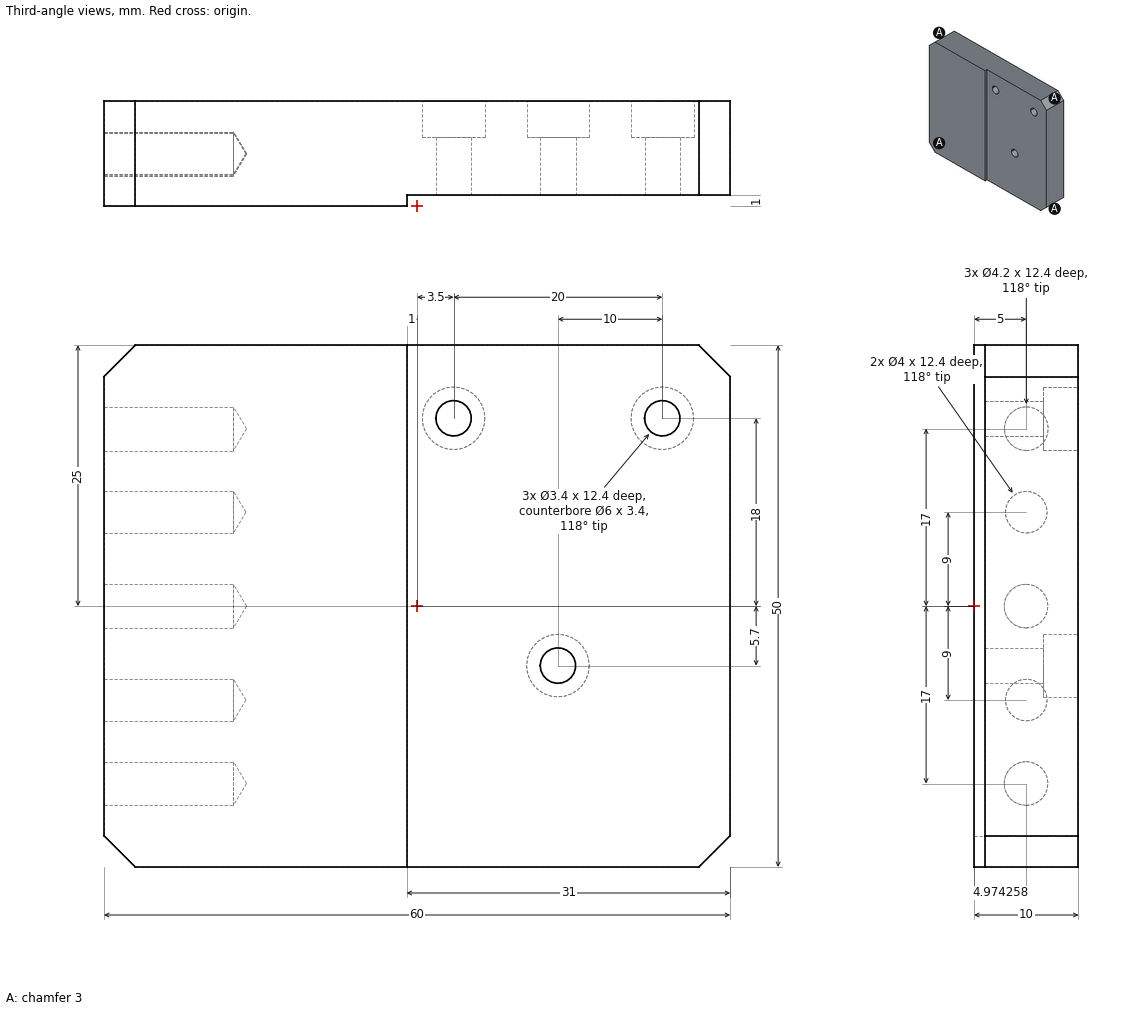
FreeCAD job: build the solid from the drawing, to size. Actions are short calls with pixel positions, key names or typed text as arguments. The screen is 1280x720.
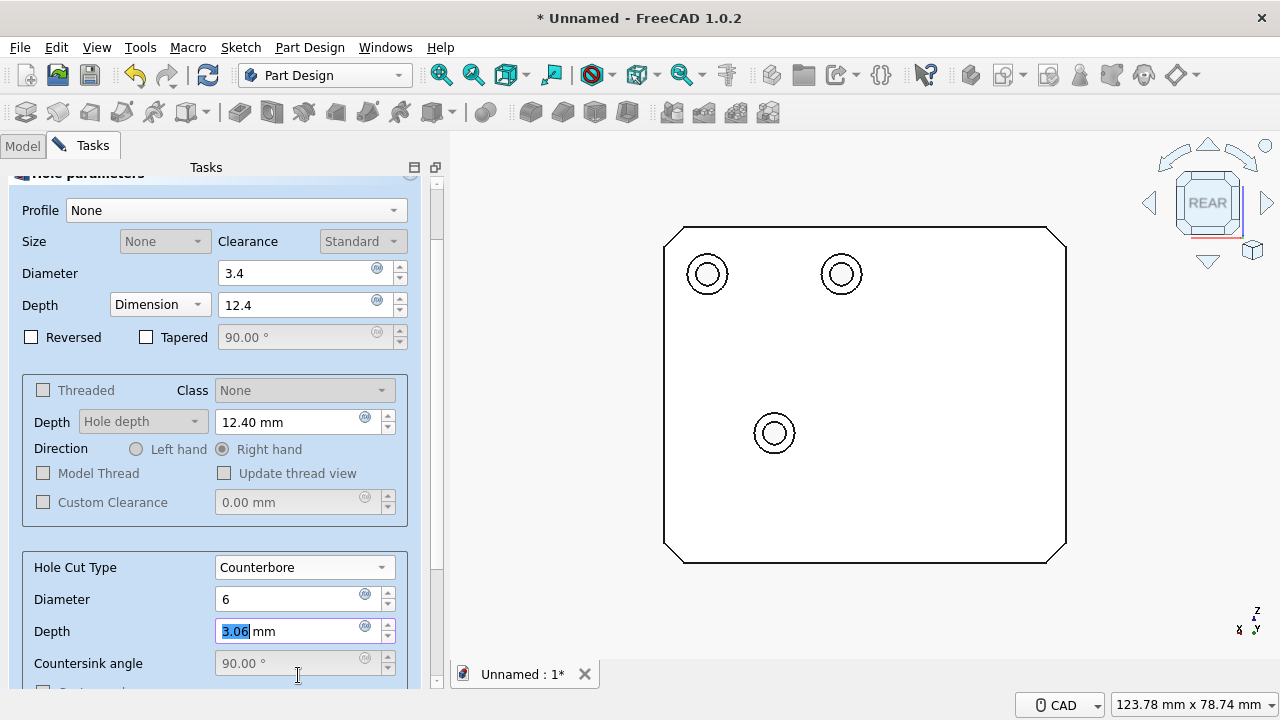
text(3.4)
key(Tab)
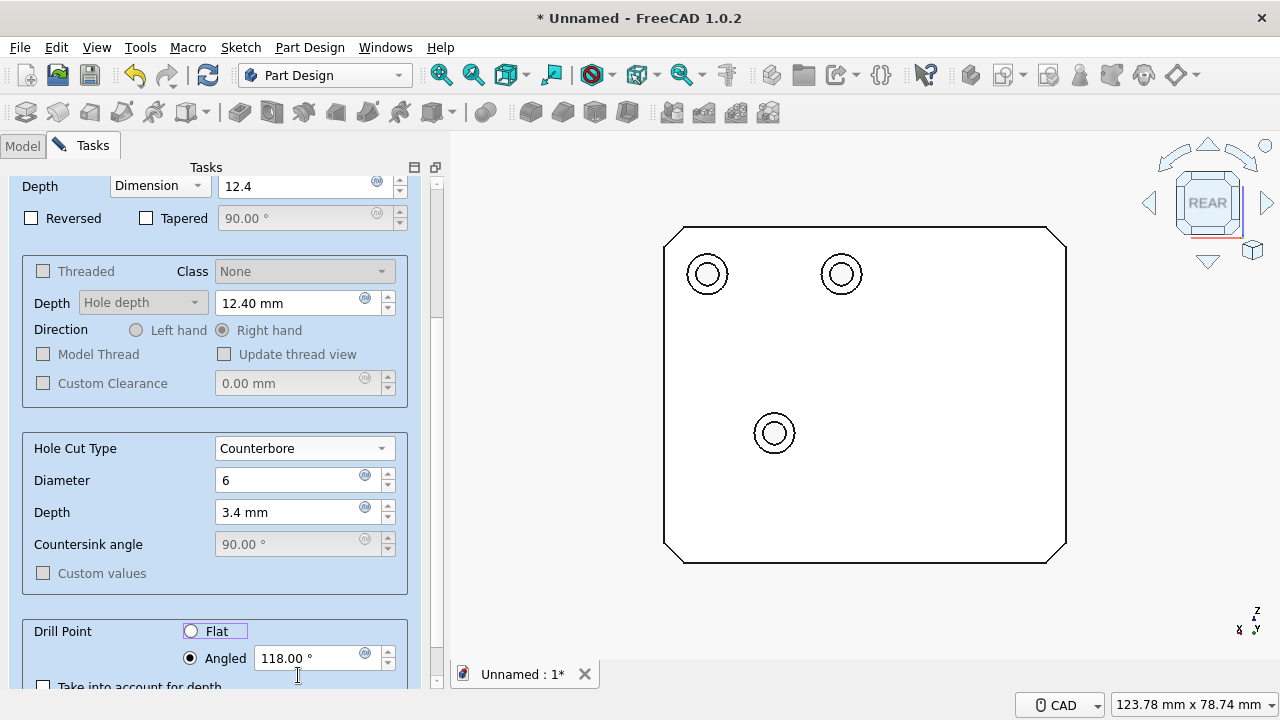
scroll(437, 432, up, 4)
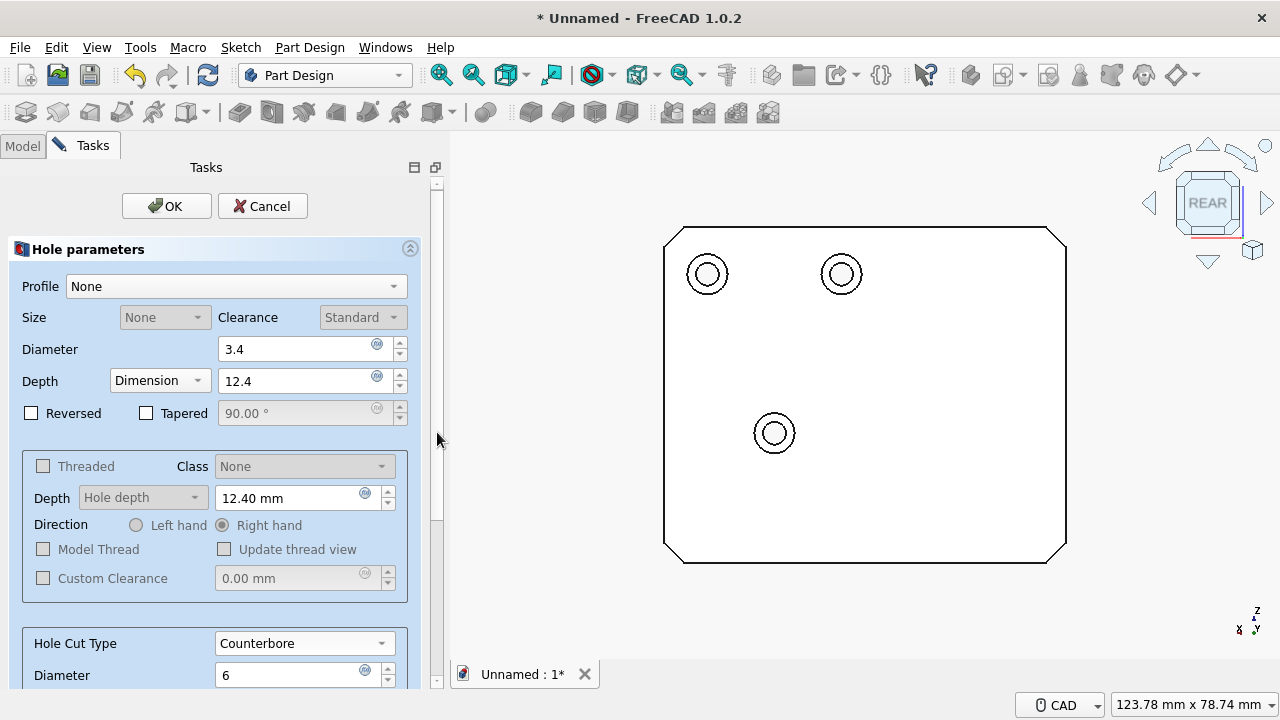
click(167, 206)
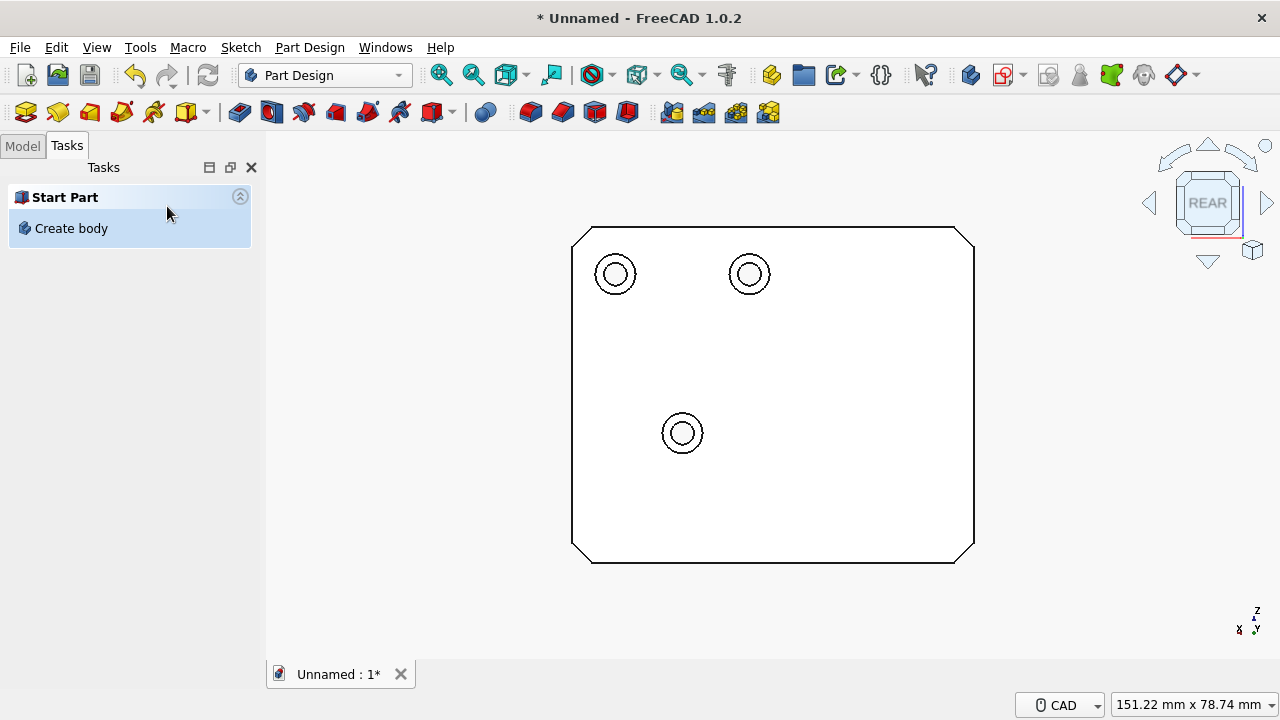
key(6)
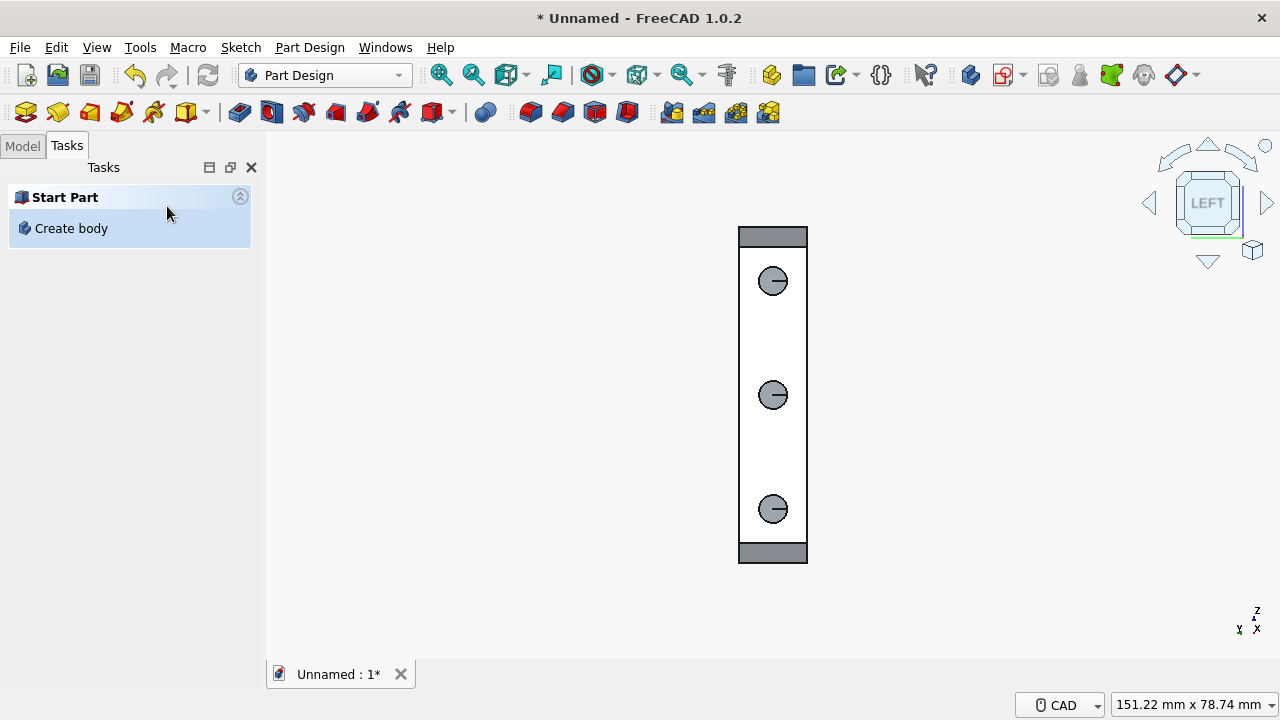
click(773, 436)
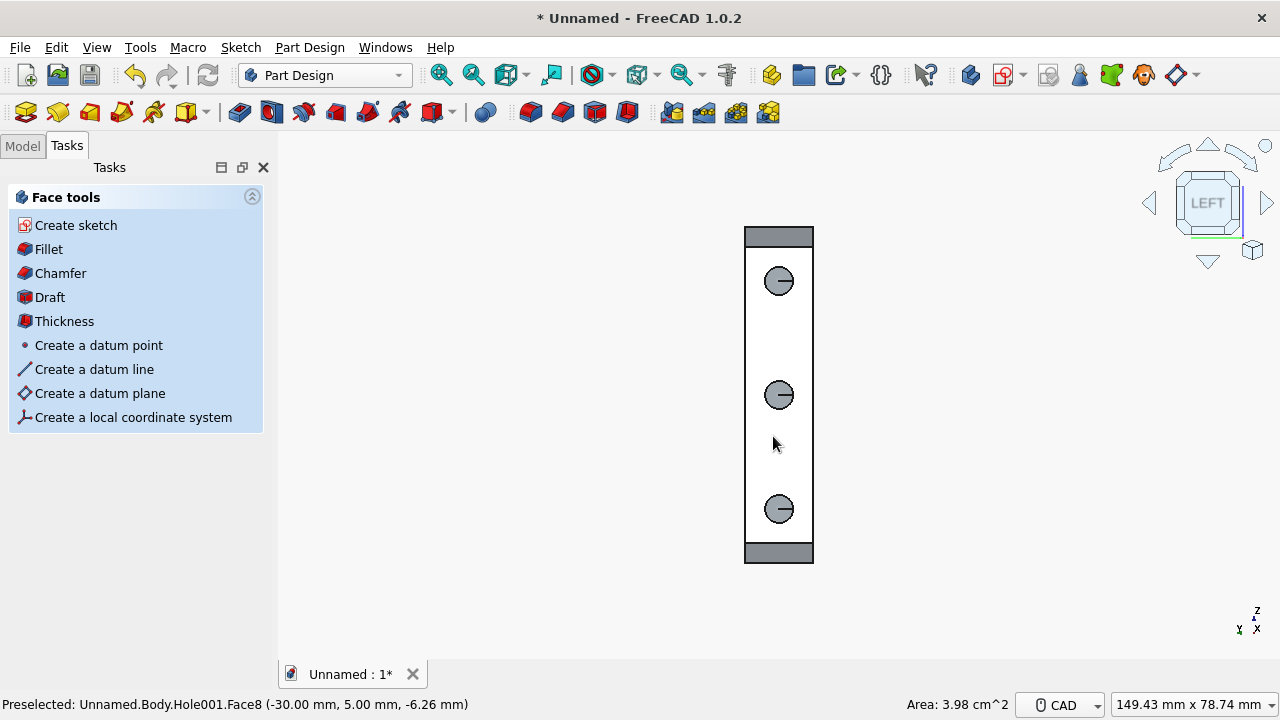
click(1004, 76)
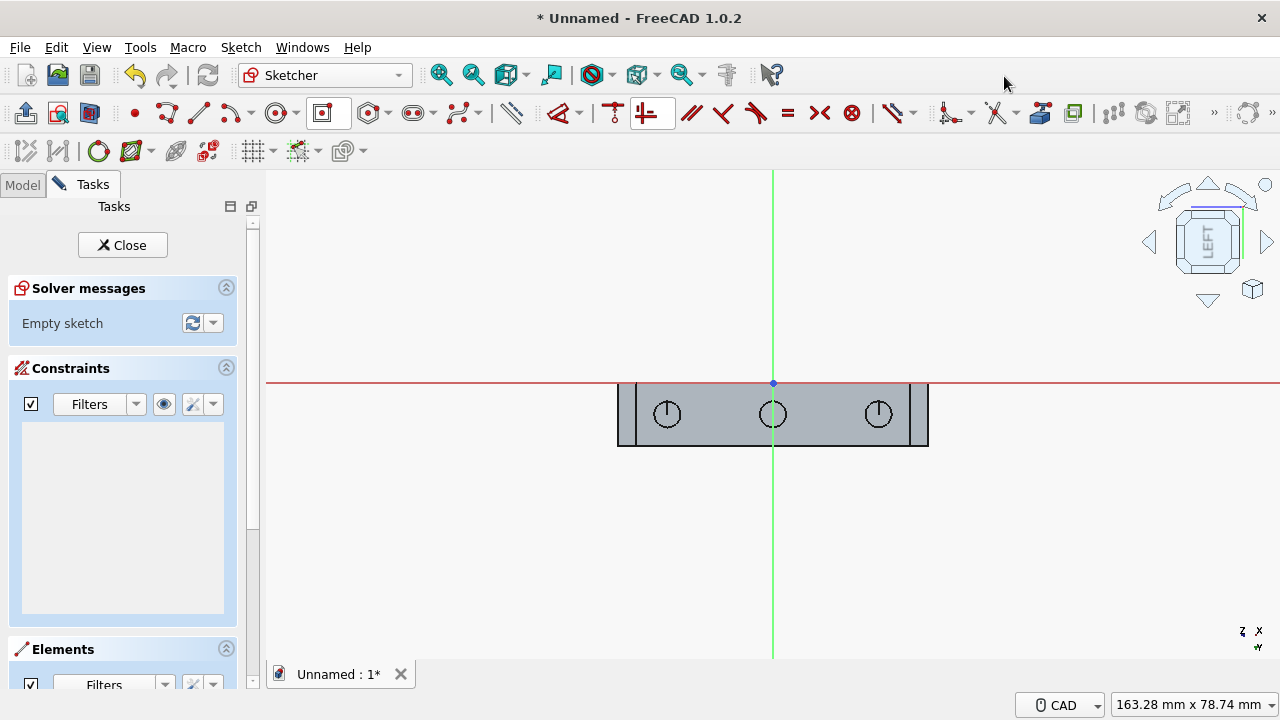
scroll(795, 402, up, 7)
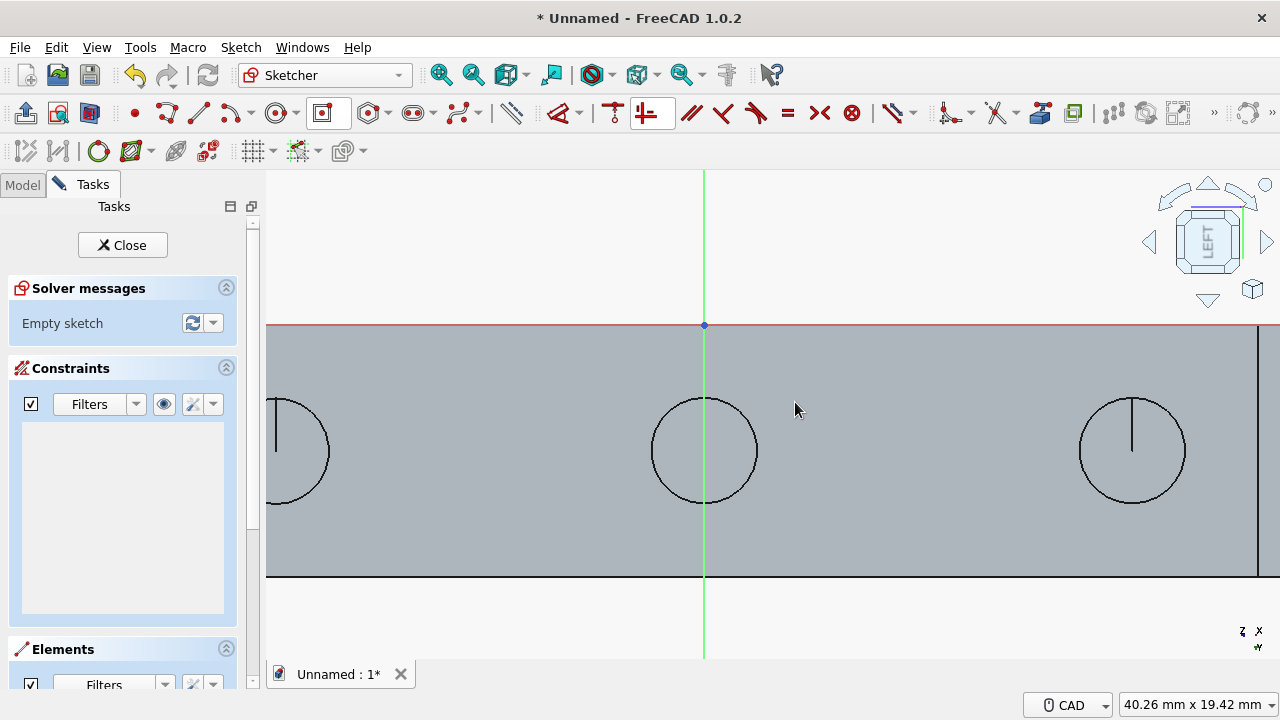
click(276, 114)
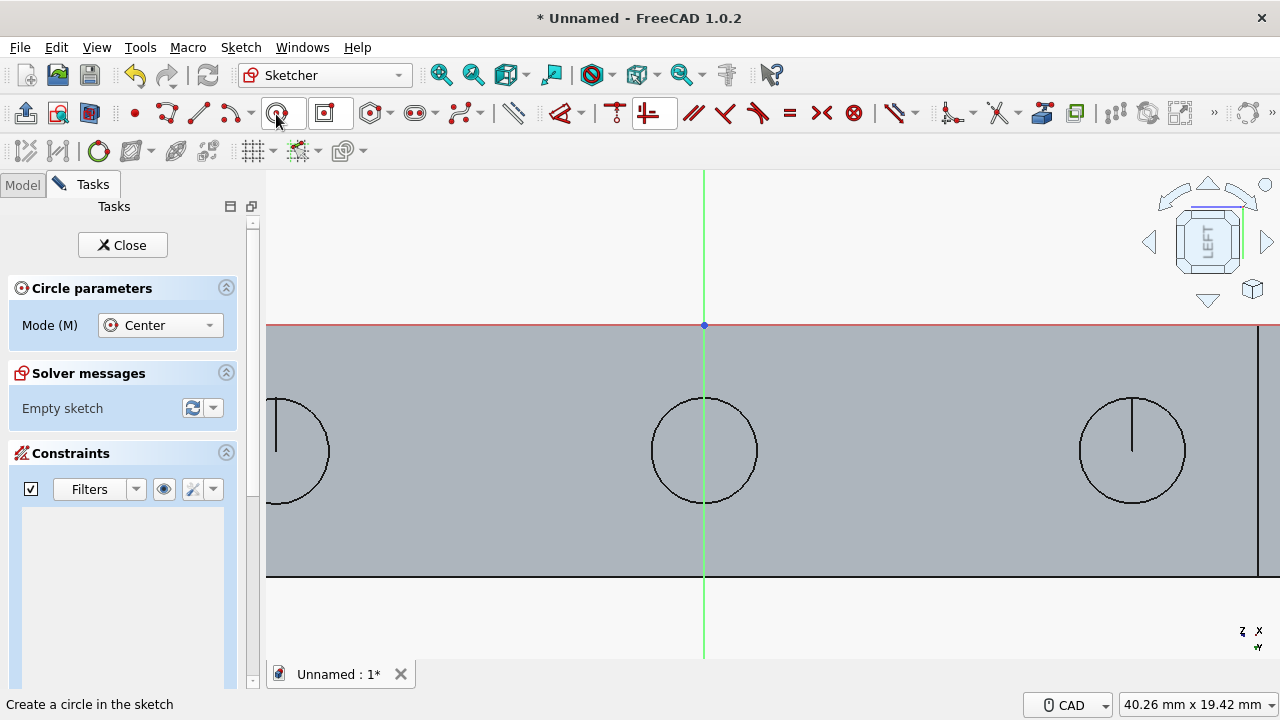
click(478, 451)
move(513, 416)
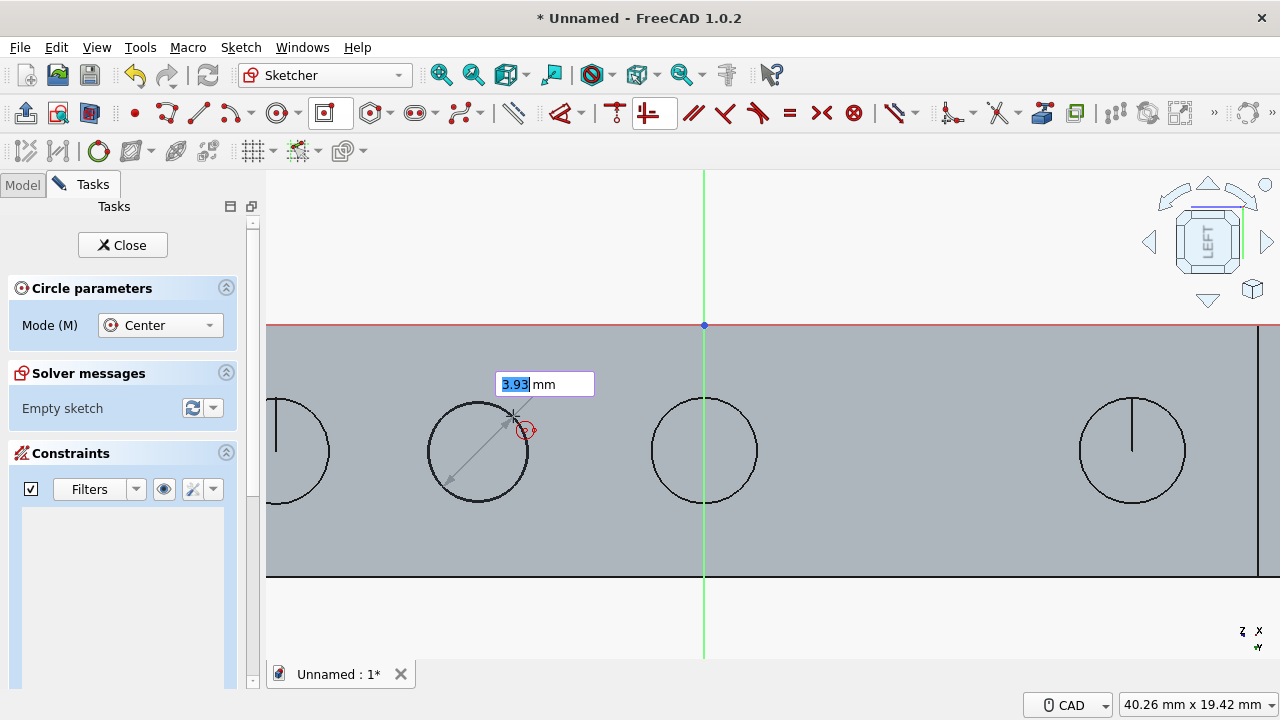
text(4)
key(Return)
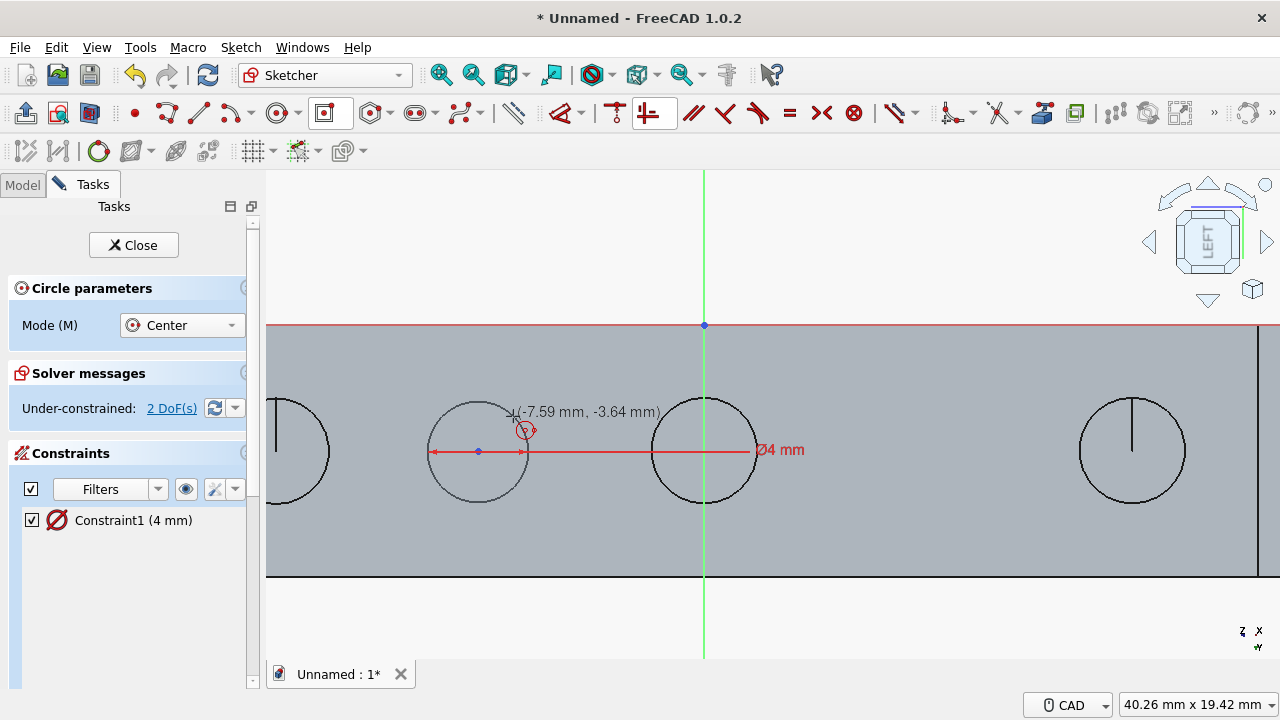
click(931, 451)
move(966, 416)